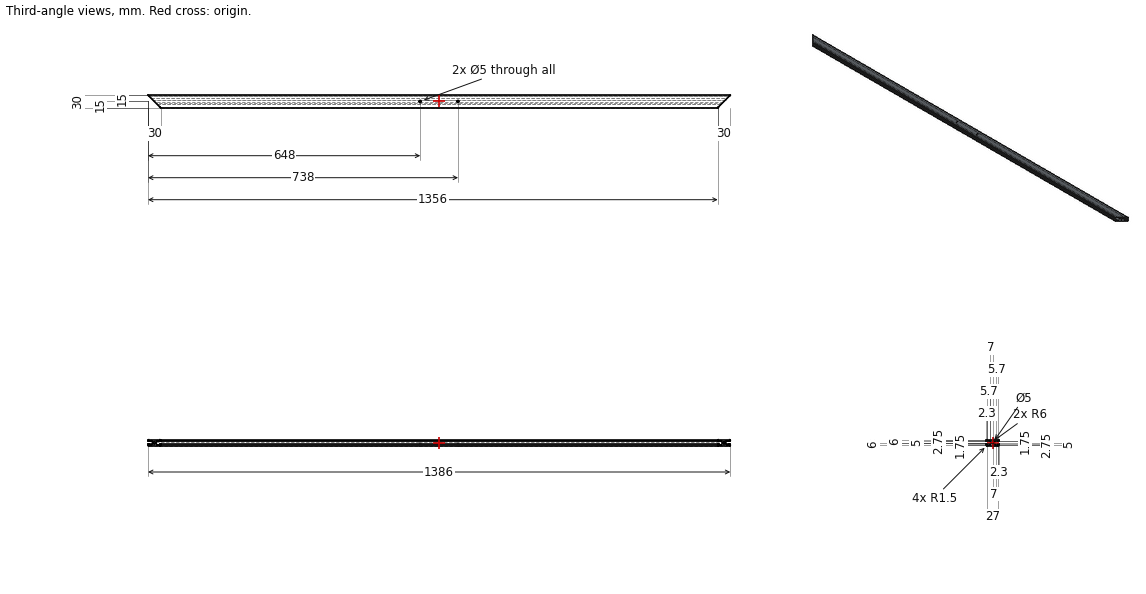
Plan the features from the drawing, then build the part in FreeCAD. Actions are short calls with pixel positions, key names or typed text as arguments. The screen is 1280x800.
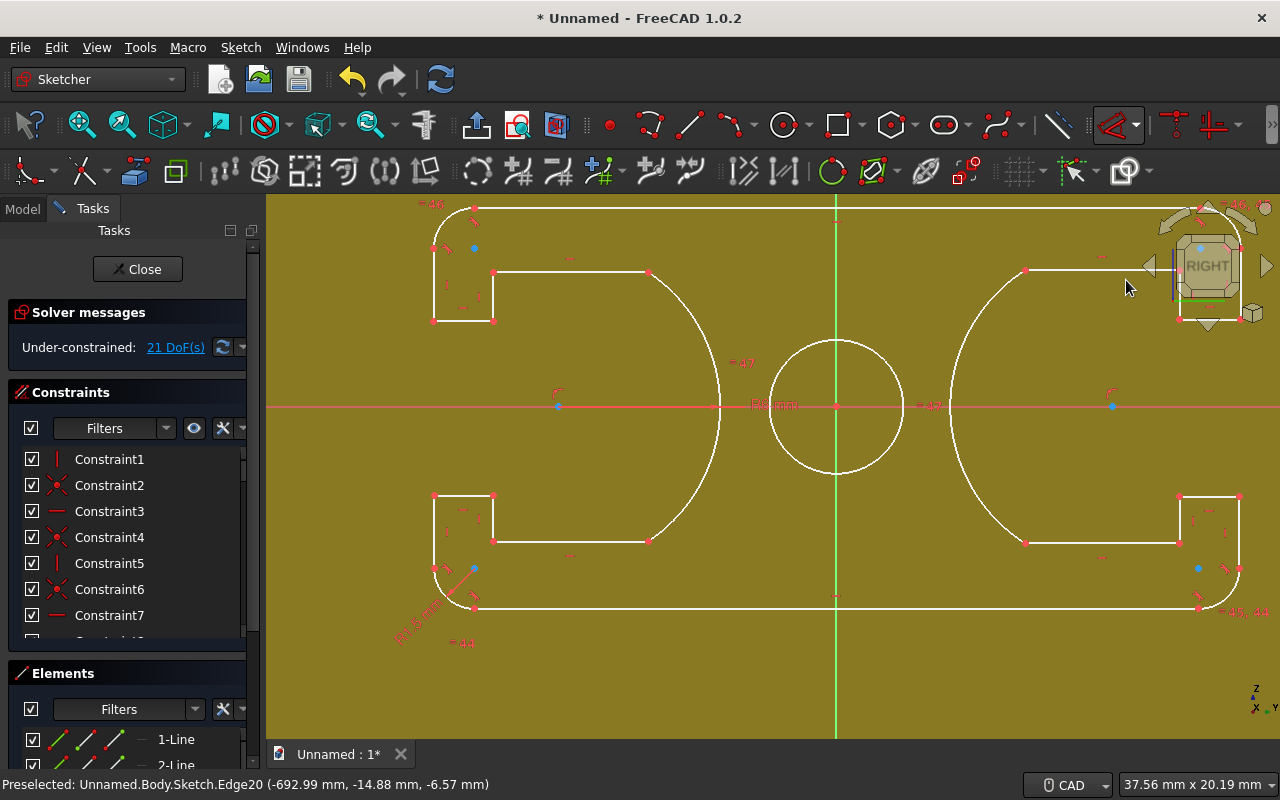
click(884, 359)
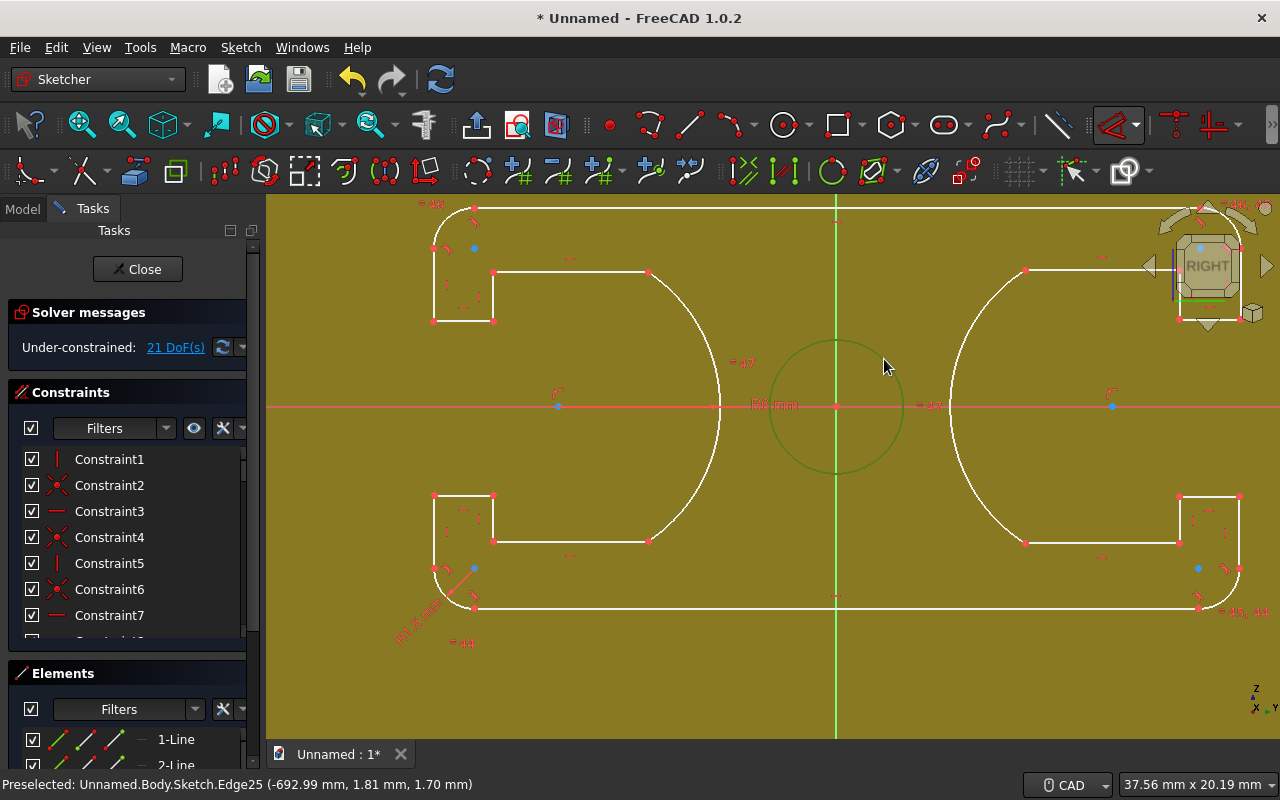
key(k)
key(o)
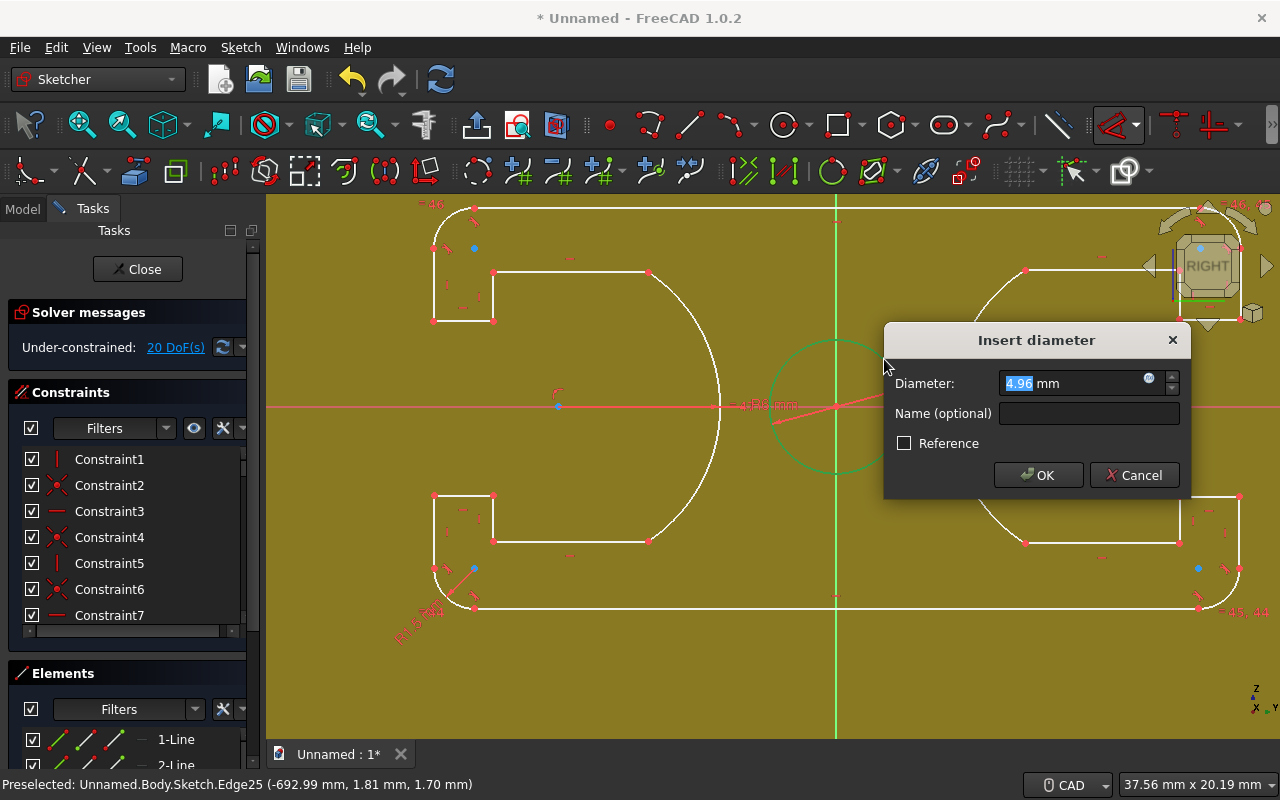
text(5)
key(Return)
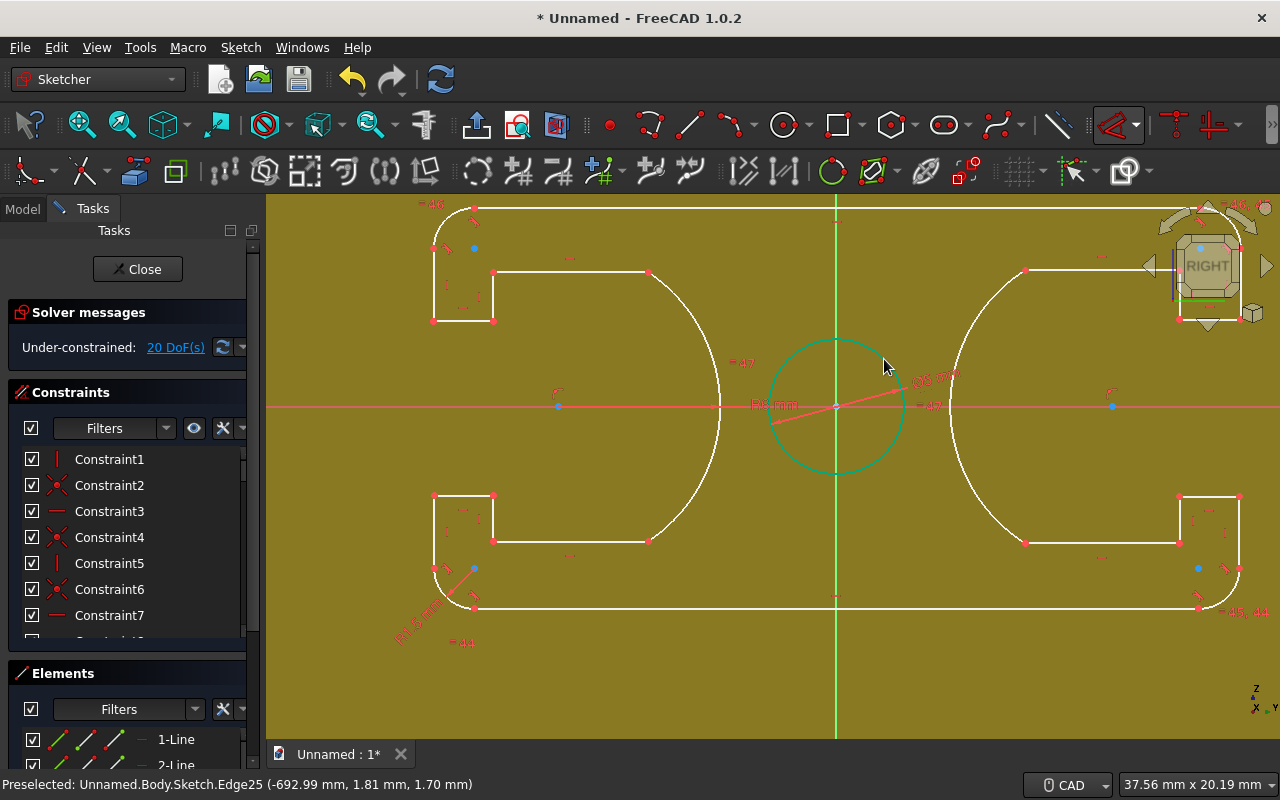
click(692, 609)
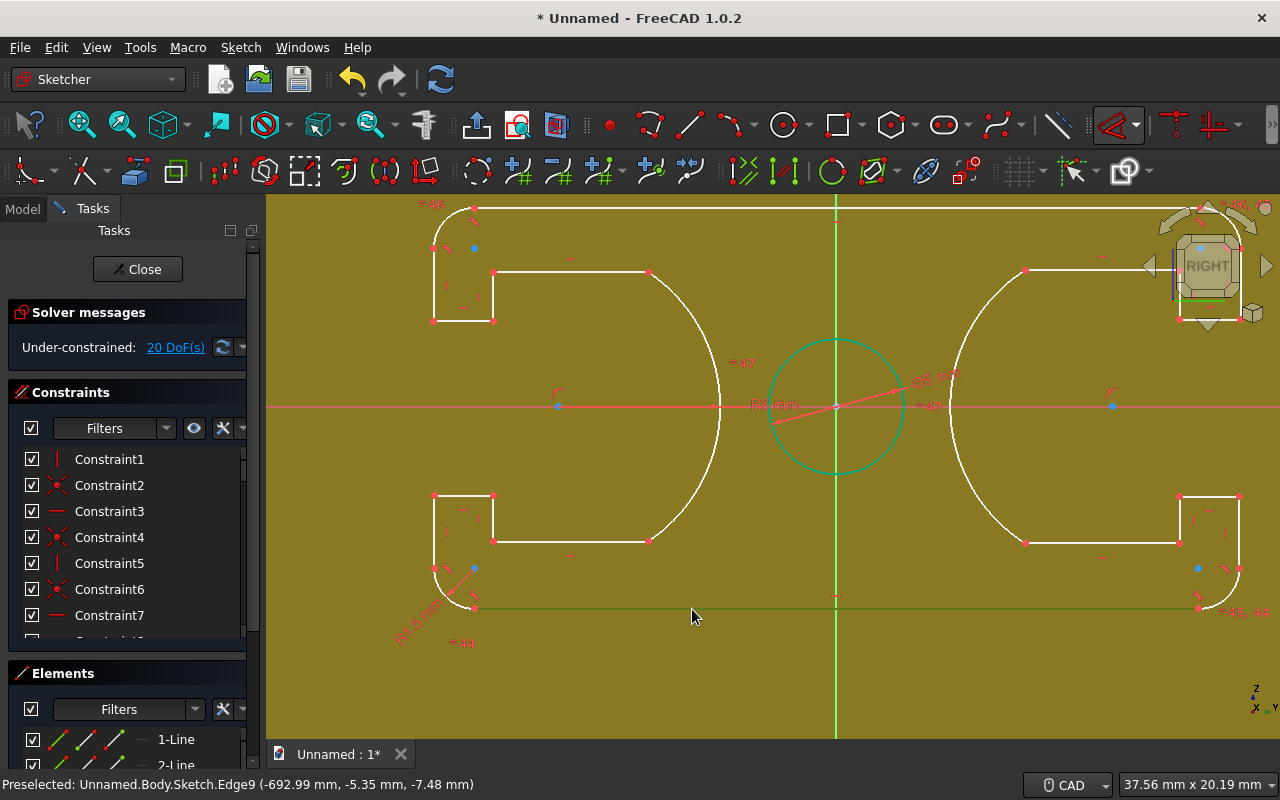
key(l)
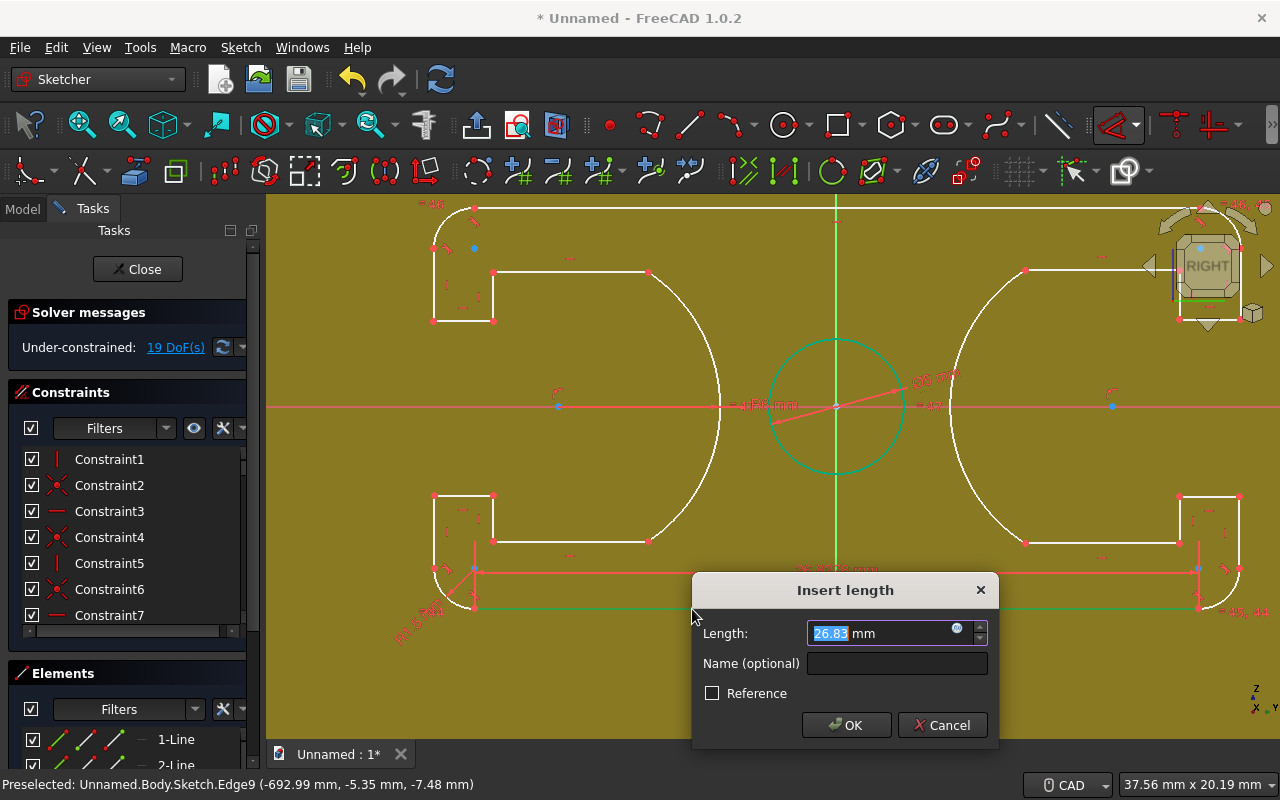
text(27)
key(Return)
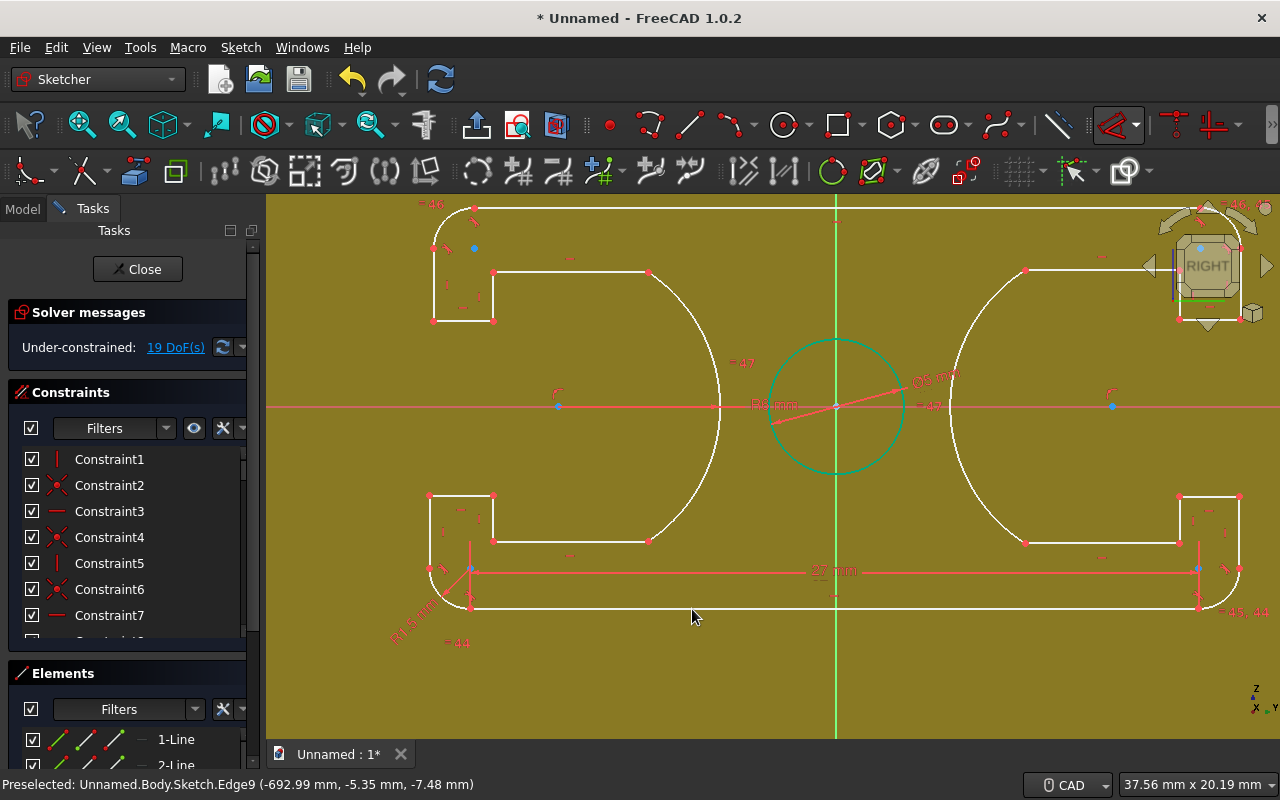
scroll(436, 588, down, 2)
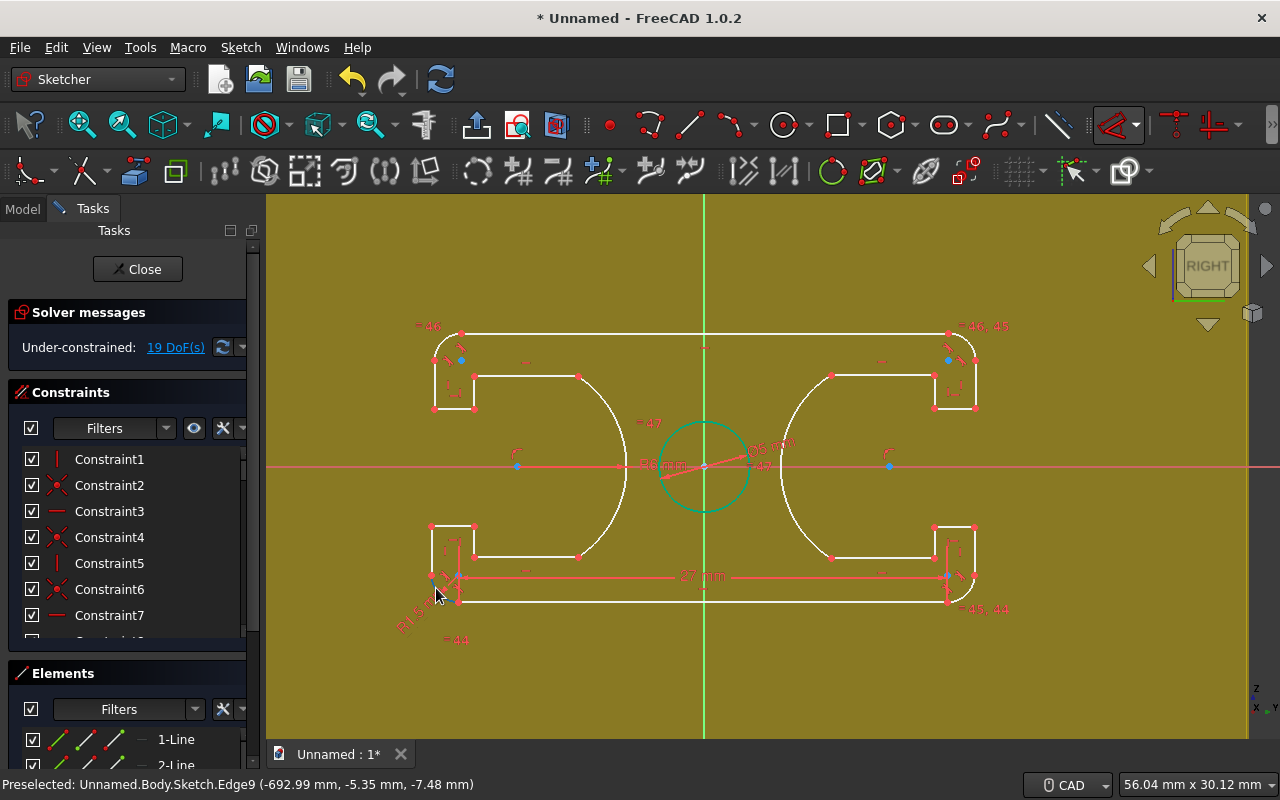
click(802, 334)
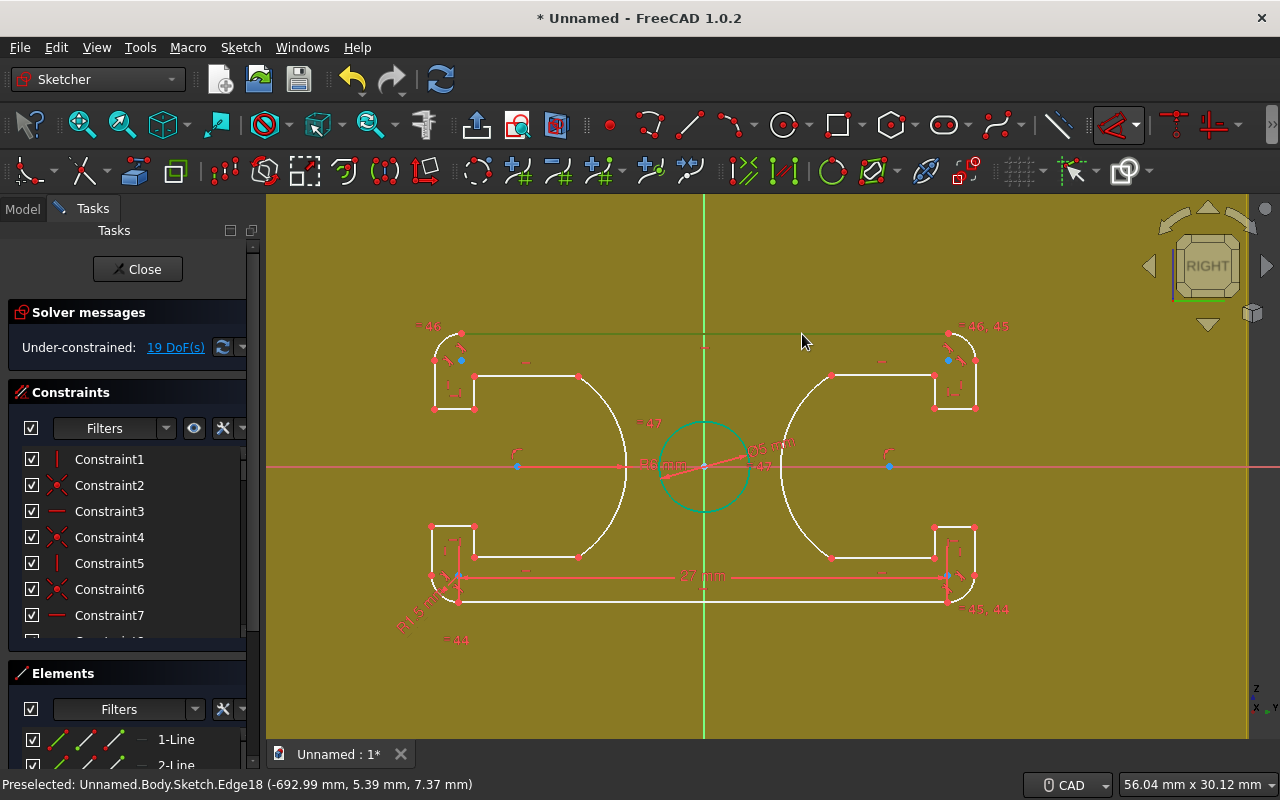
key(l)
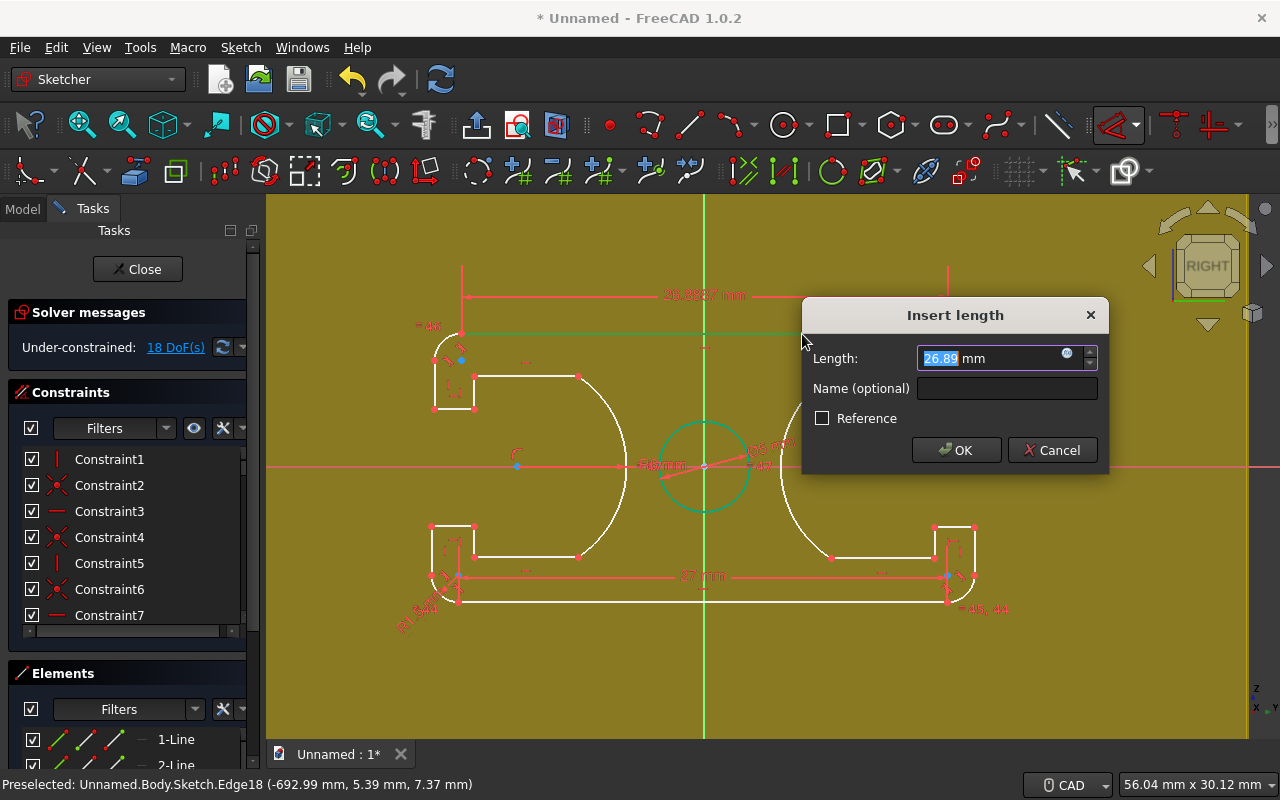
text(27)
key(Return)